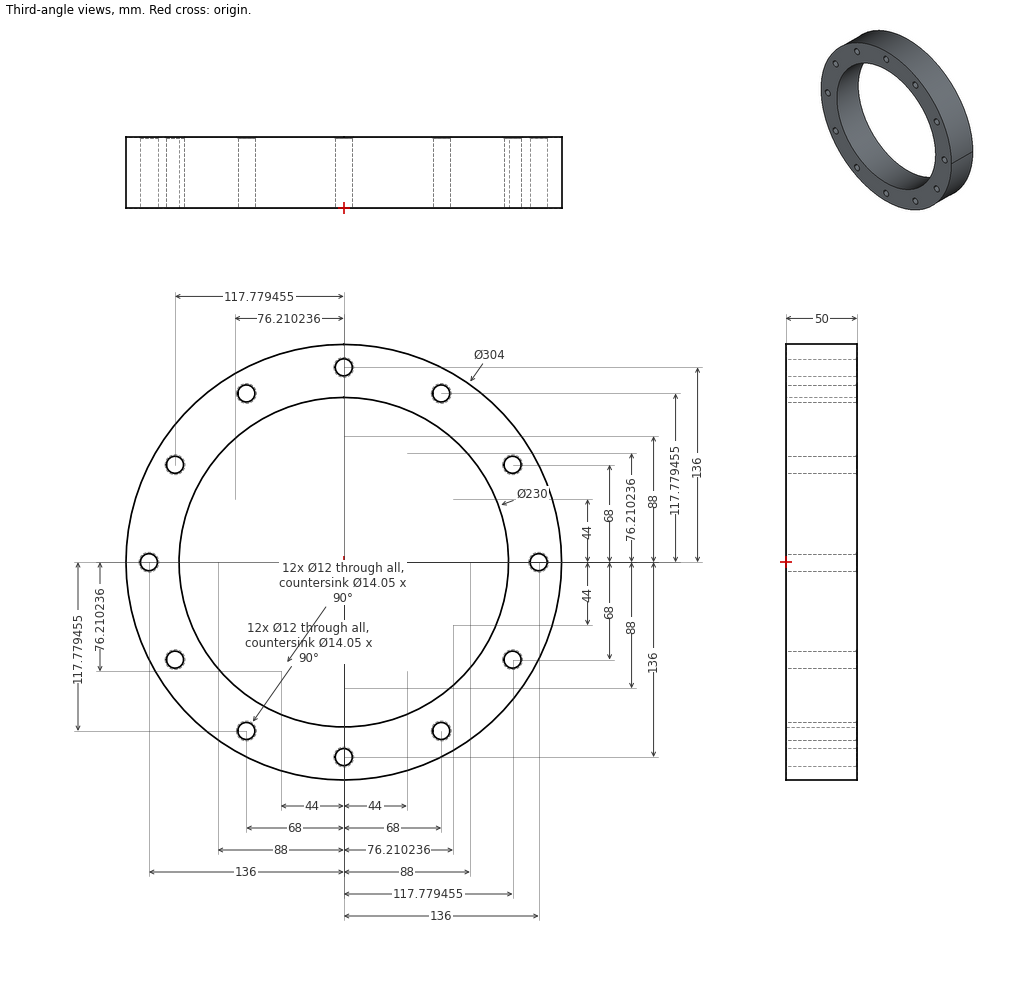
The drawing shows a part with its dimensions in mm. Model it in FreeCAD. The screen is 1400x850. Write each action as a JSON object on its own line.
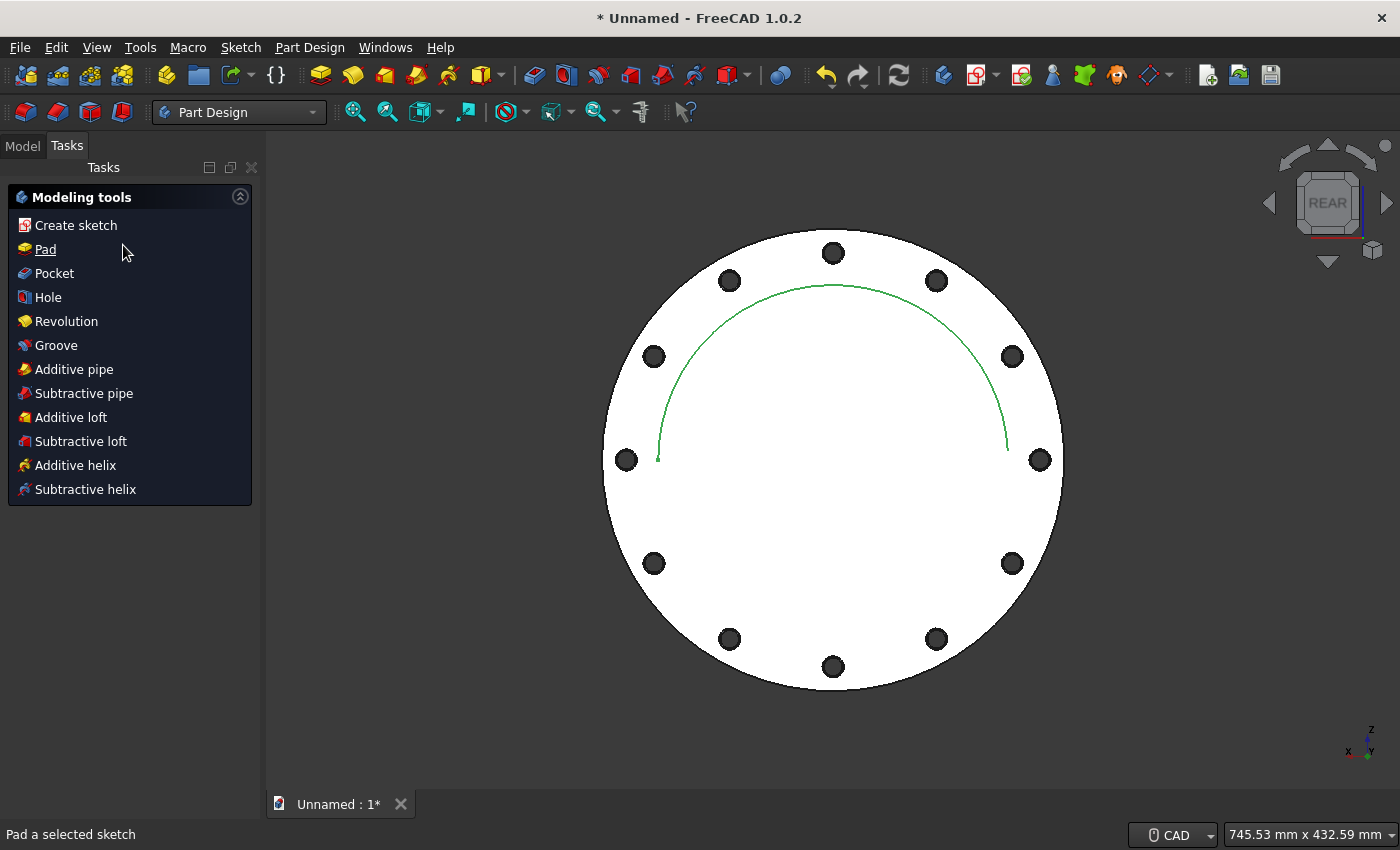
{"action": "left_click", "coordinate": [322, 76]}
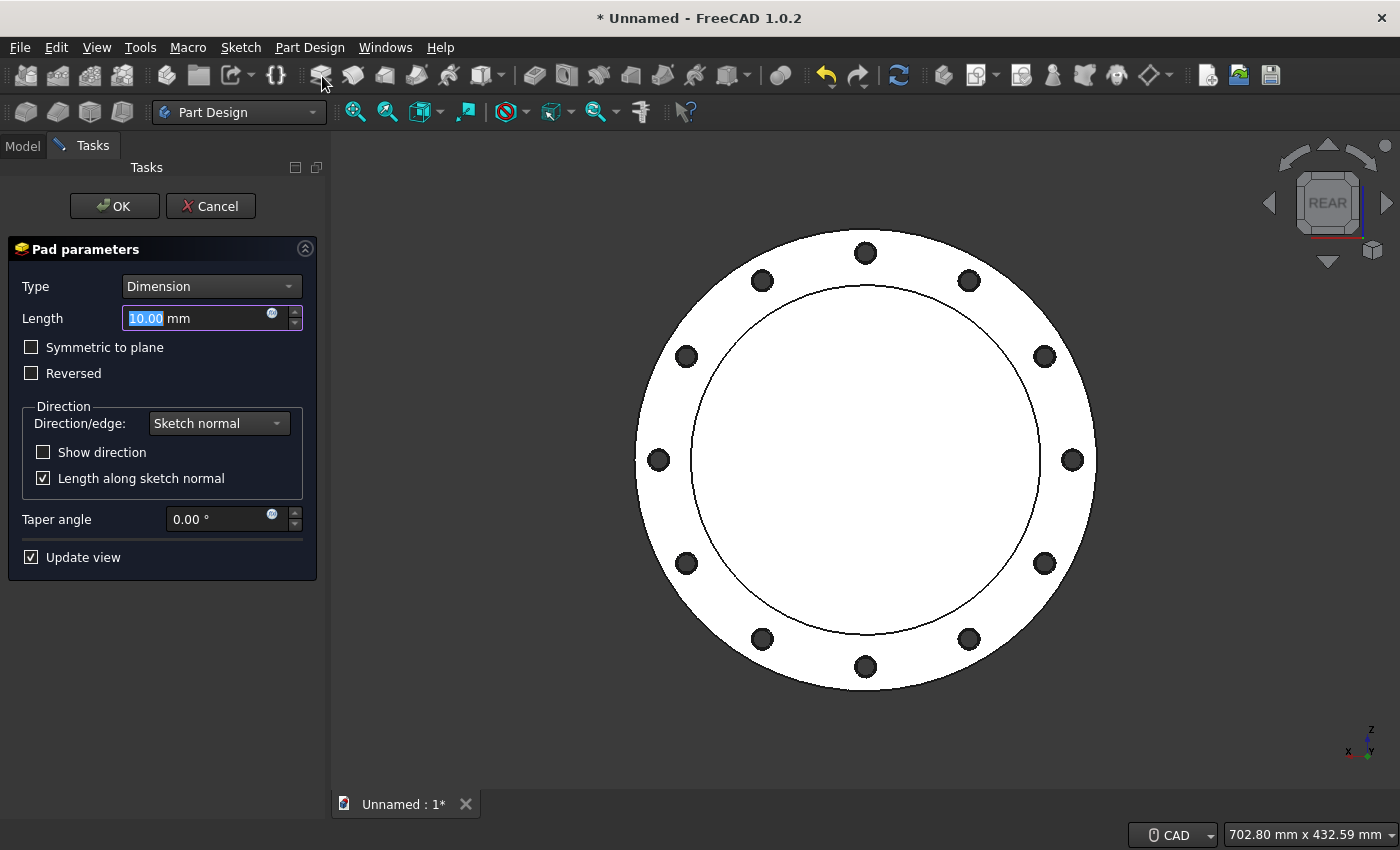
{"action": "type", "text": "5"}
{"action": "key", "text": "Tab"}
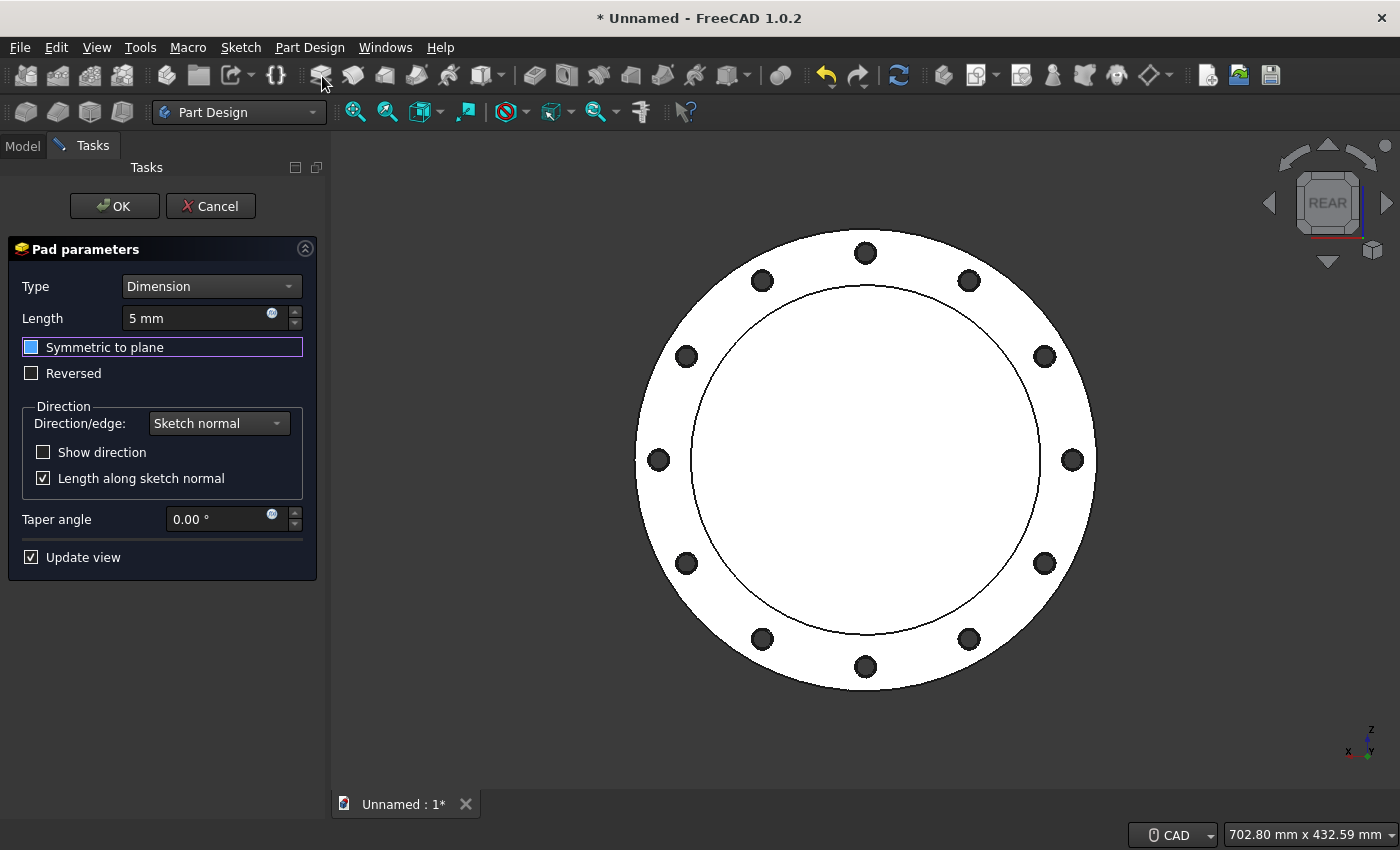
{"action": "left_click", "coordinate": [115, 206]}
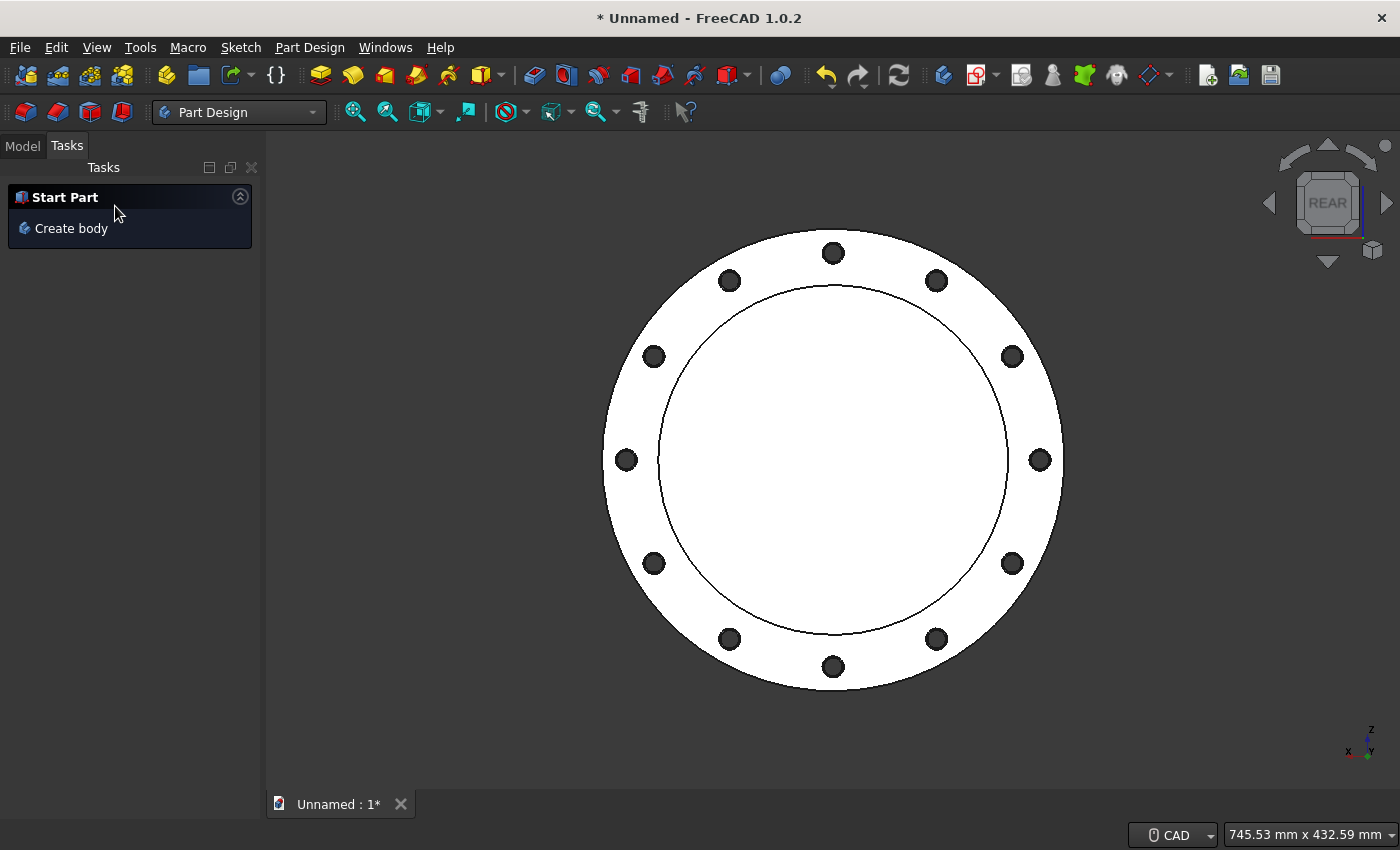
{"action": "left_click", "coordinate": [833, 459]}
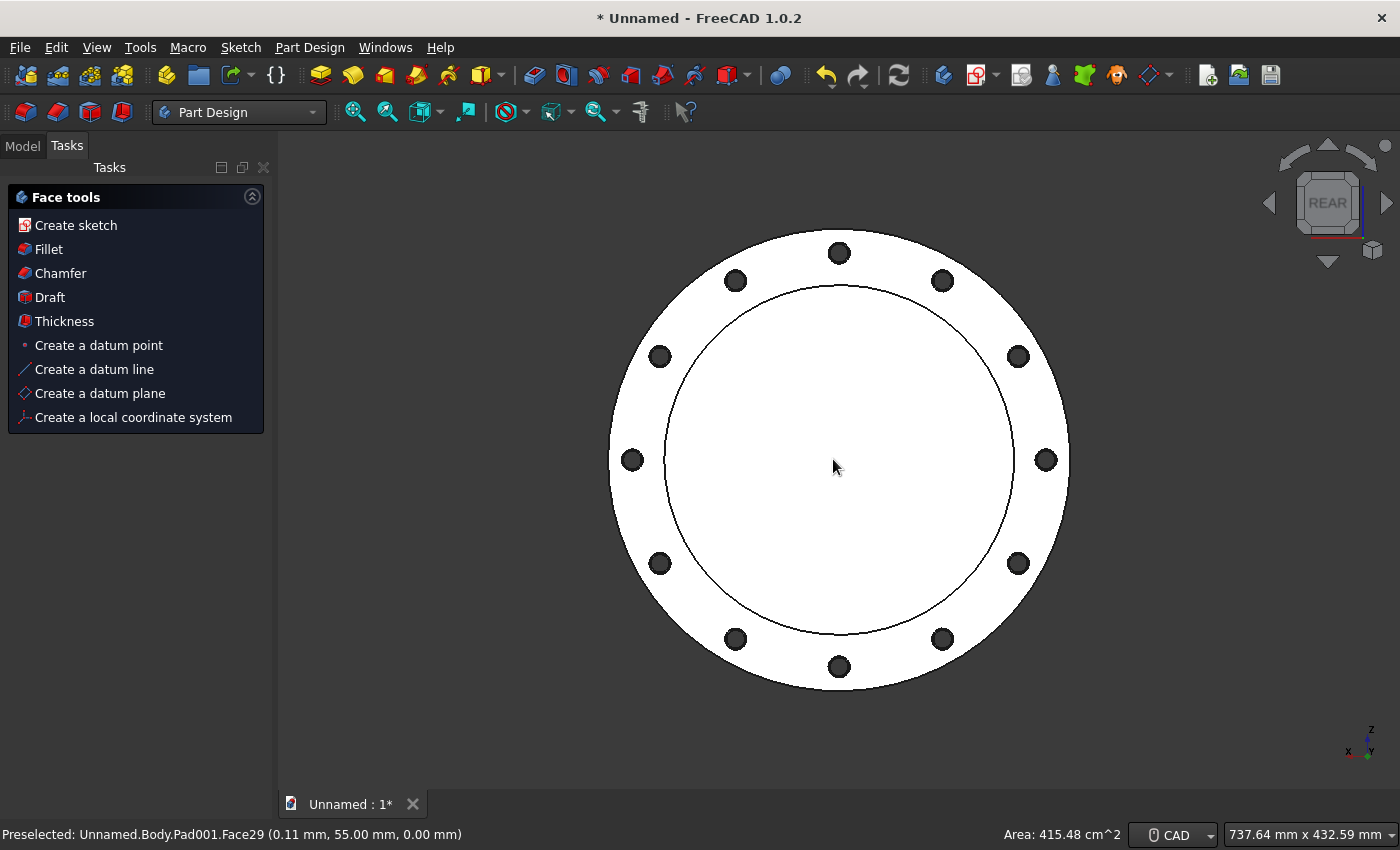
{"action": "left_click", "coordinate": [976, 76]}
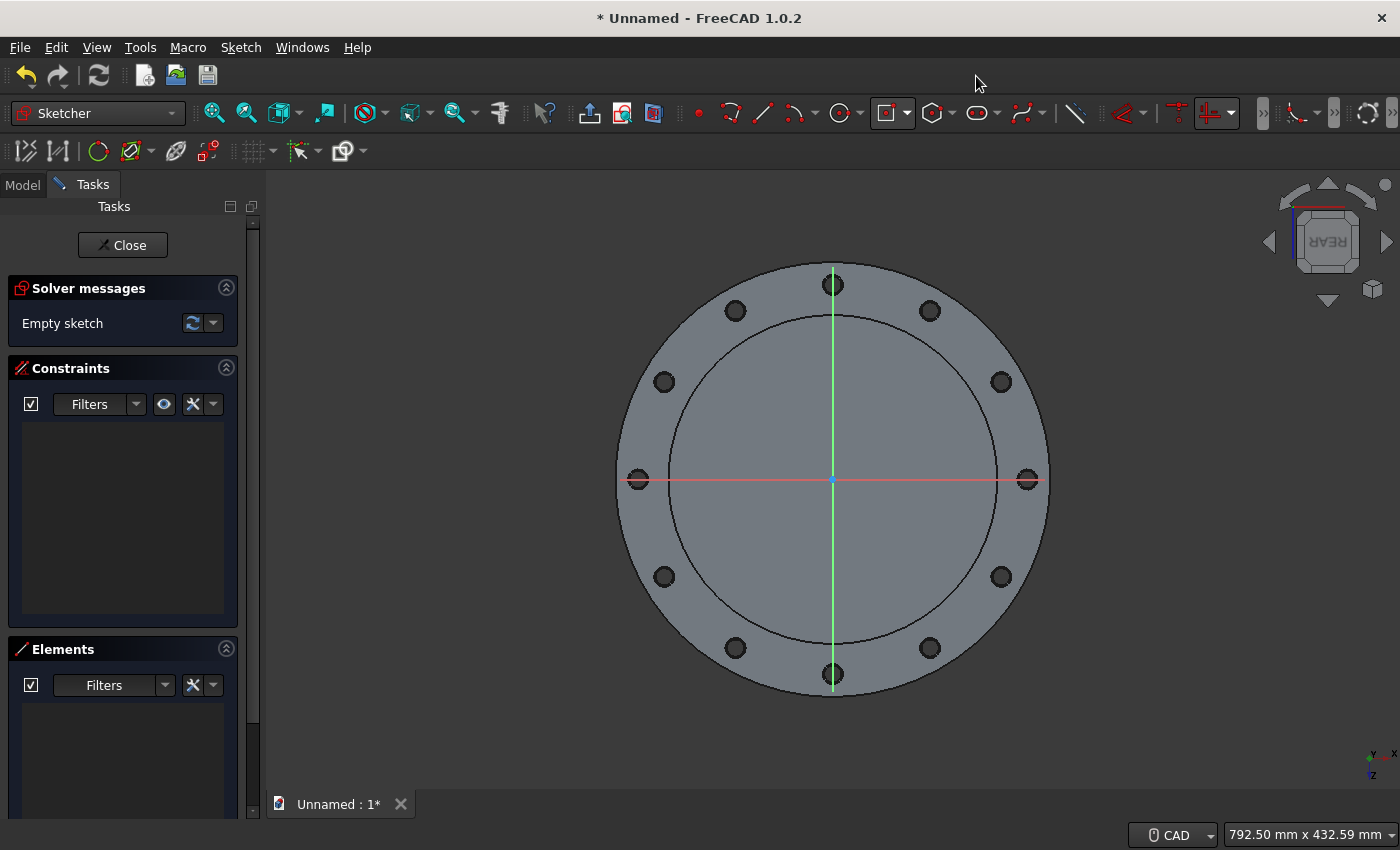
{"action": "scroll", "coordinate": [972, 479], "scroll_direction": "up", "scroll_amount": 2}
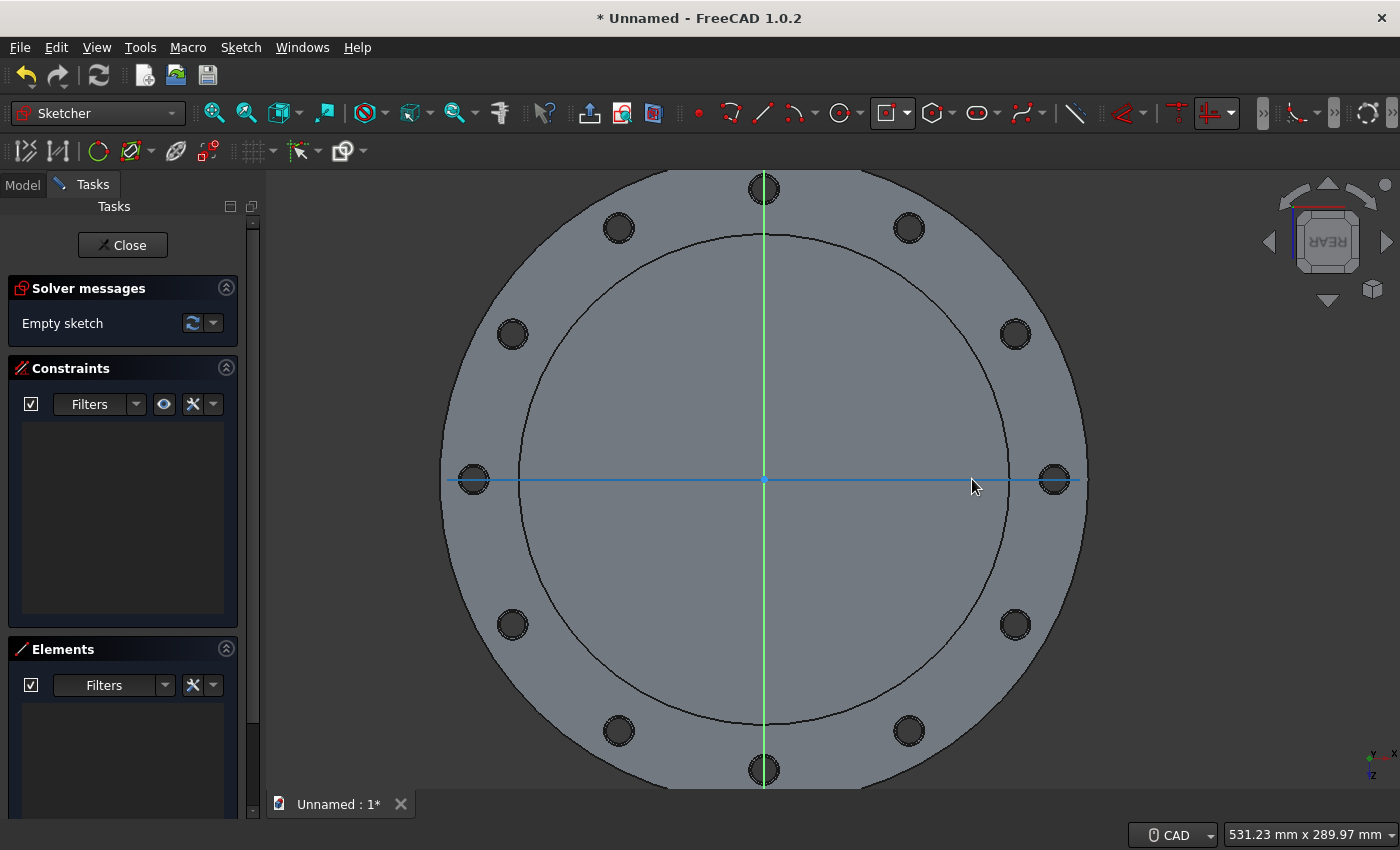
{"action": "left_click", "coordinate": [840, 114]}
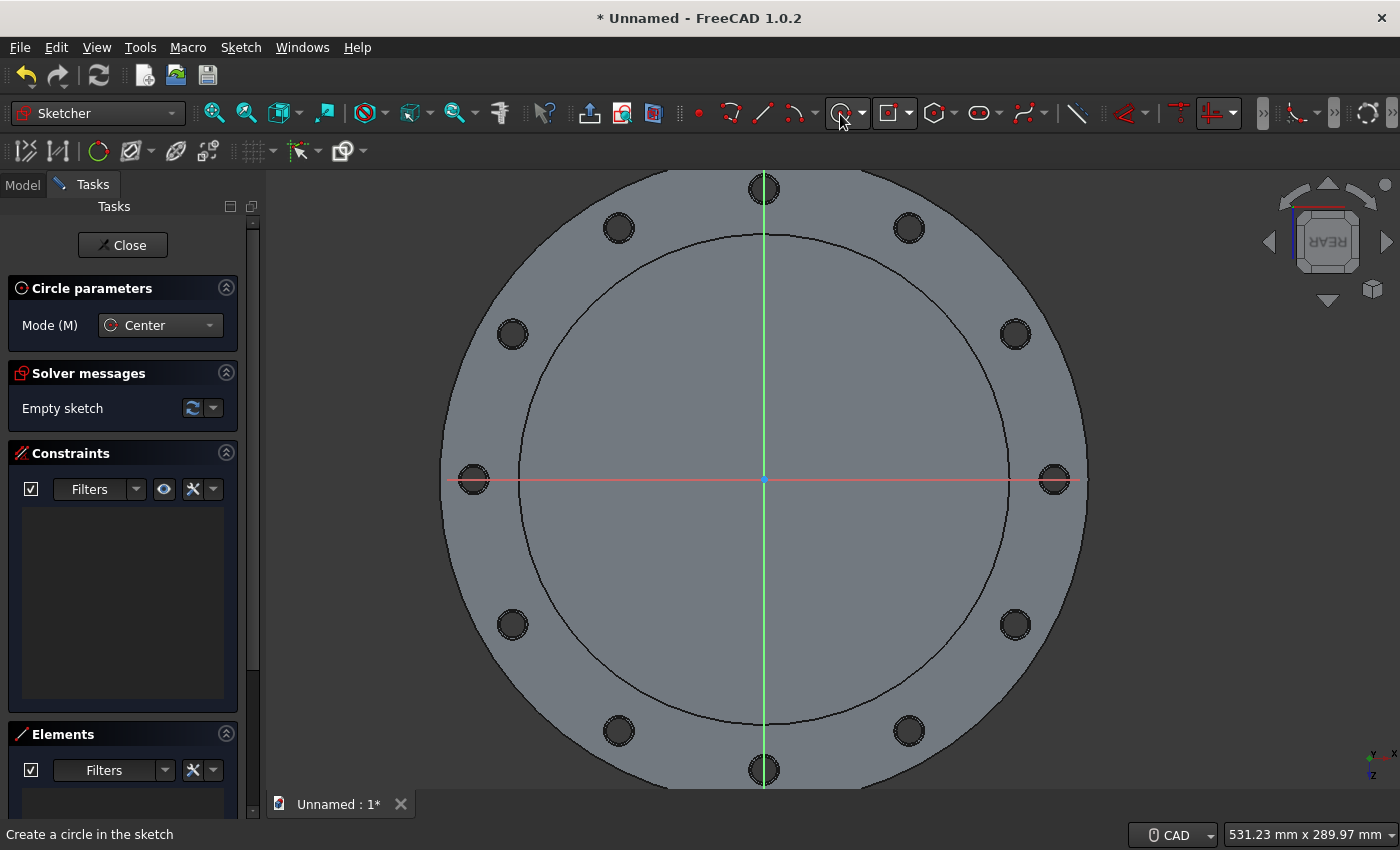
{"action": "scroll", "coordinate": [670, 317], "scroll_direction": "up", "scroll_amount": 3}